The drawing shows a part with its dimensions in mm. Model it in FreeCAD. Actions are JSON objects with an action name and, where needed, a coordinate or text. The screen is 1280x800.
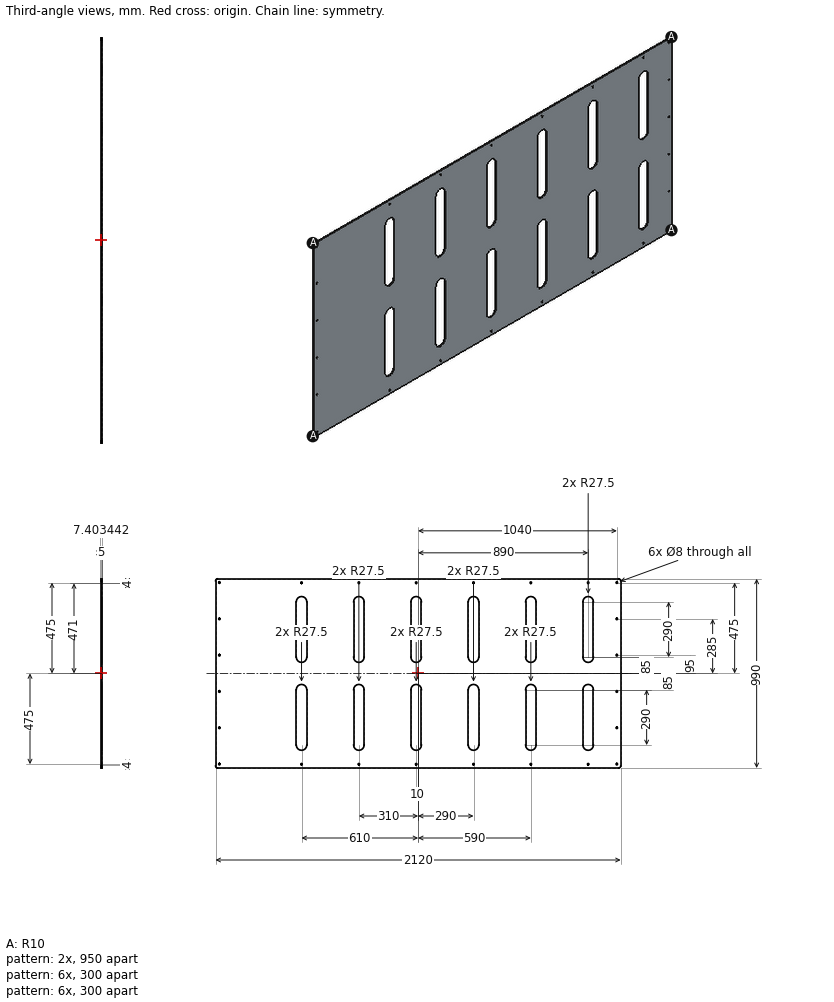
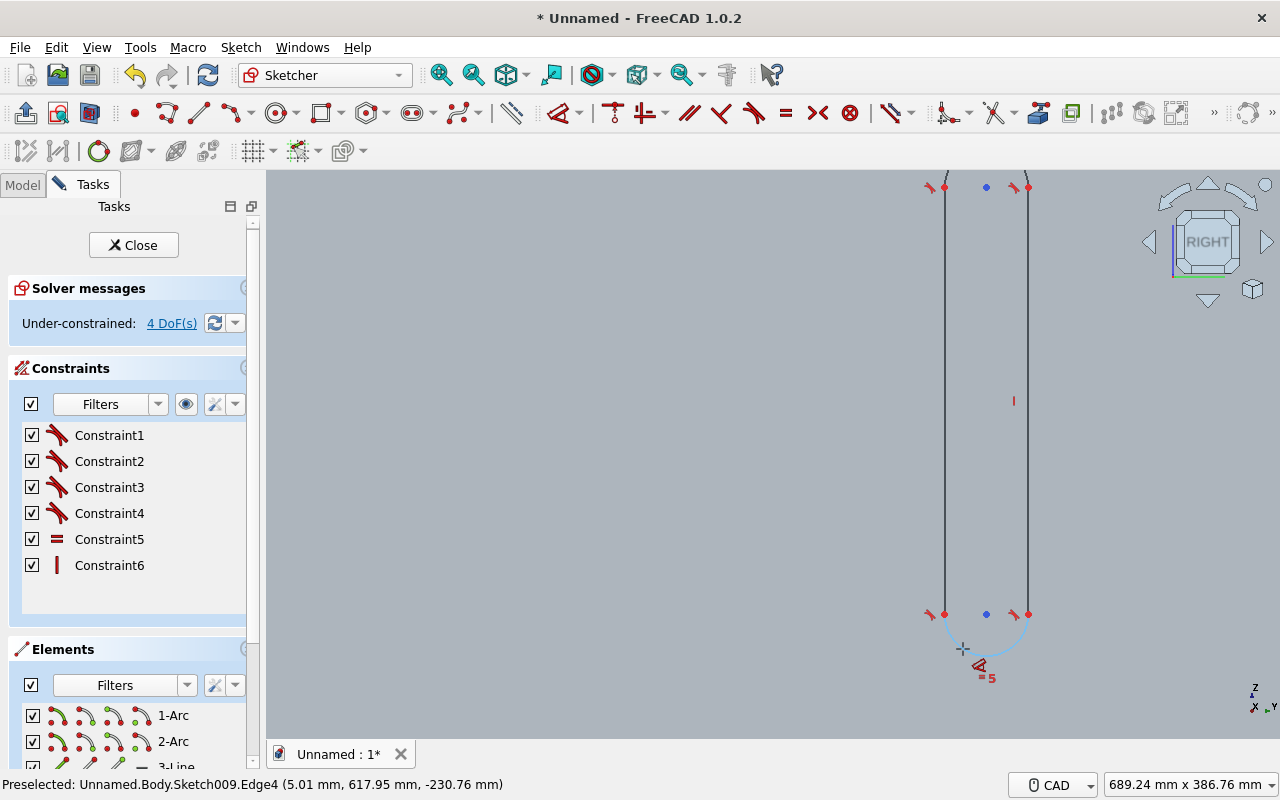
{"action": "left_click", "coordinate": [962, 648]}
{"action": "left_click", "coordinate": [943, 674]}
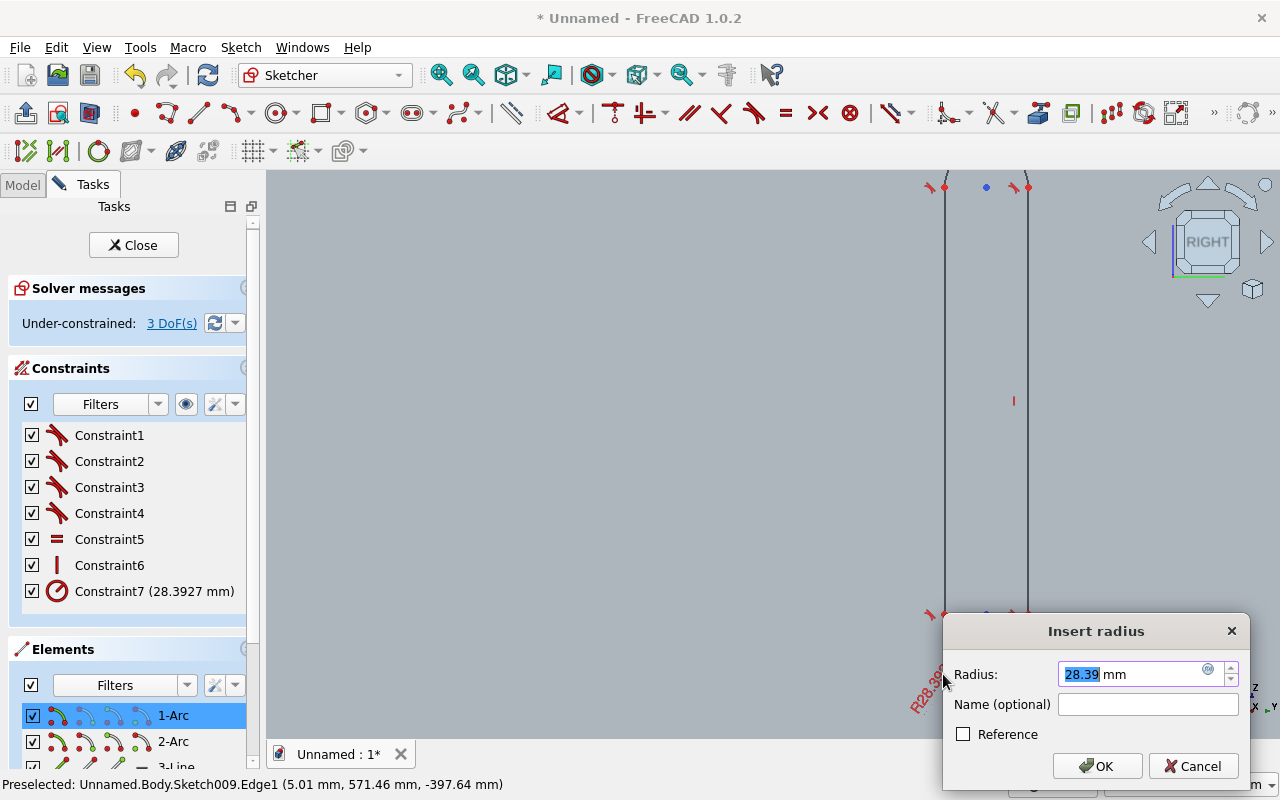
{"action": "type", "text": "27.5"}
{"action": "key", "text": "Return"}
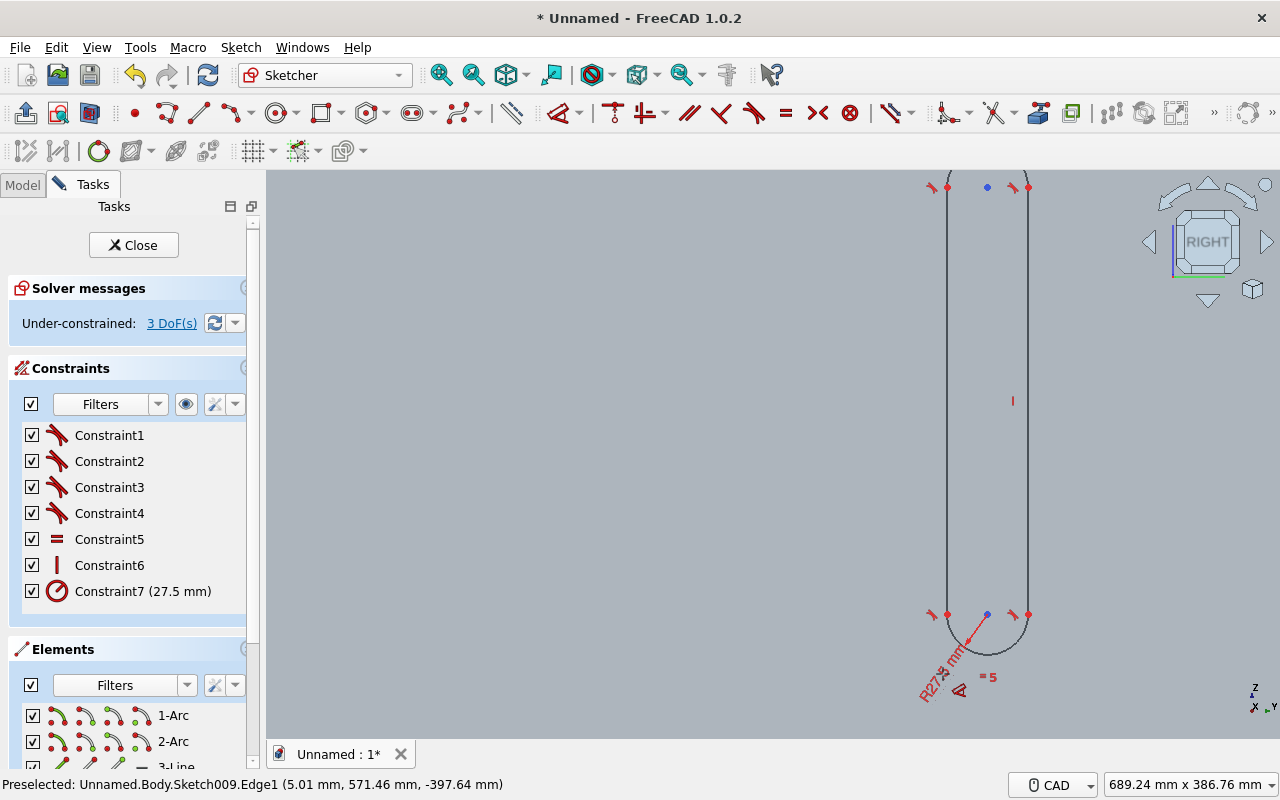
{"action": "left_click", "coordinate": [947, 486]}
{"action": "left_click", "coordinate": [981, 406]}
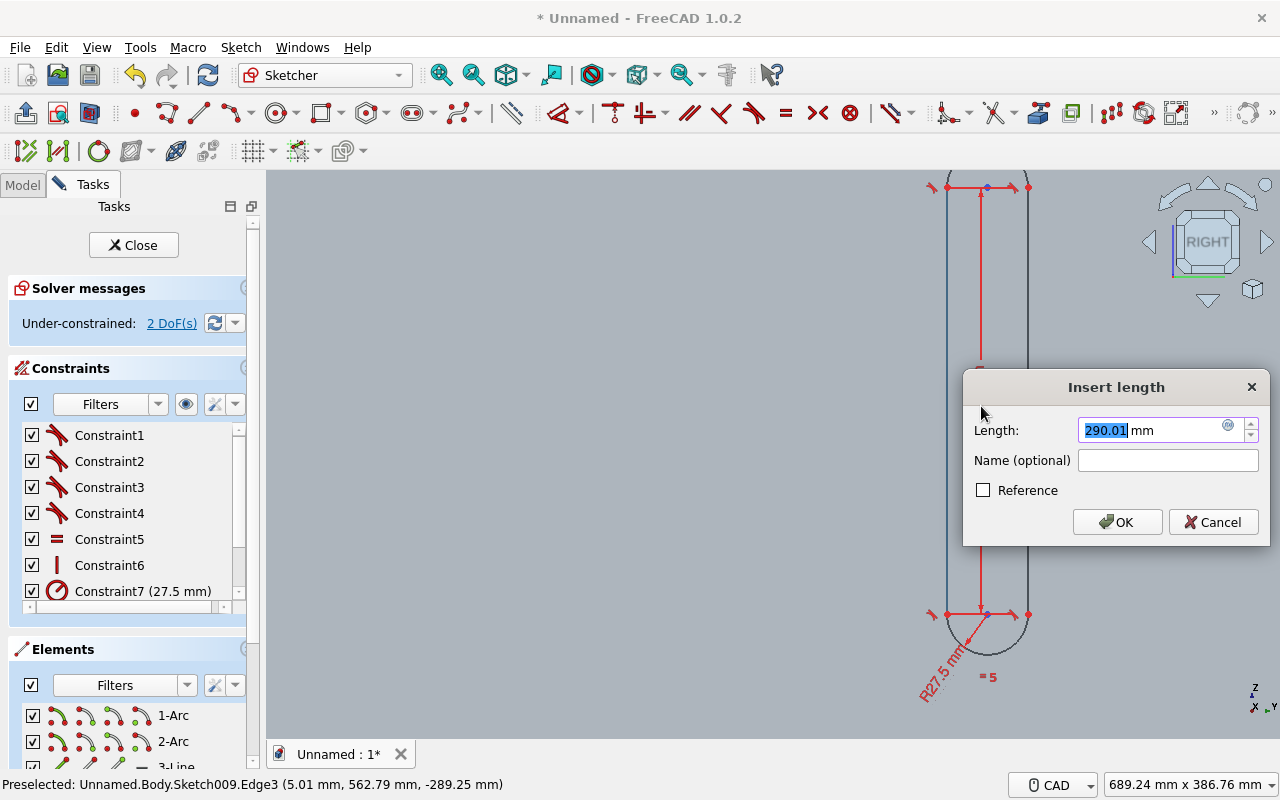
{"action": "type", "text": "290"}
{"action": "key", "text": "Return"}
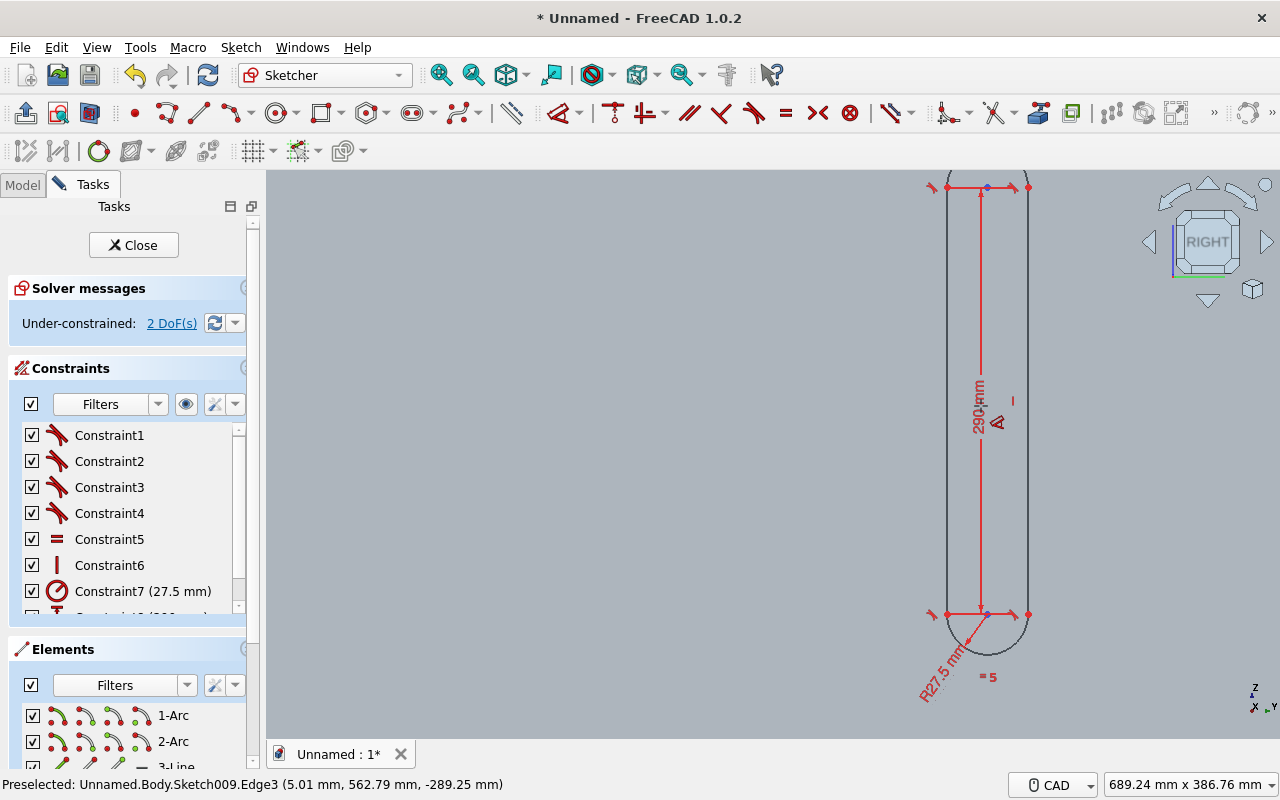
{"action": "scroll", "coordinate": [971, 652], "scroll_direction": "down", "scroll_amount": 2}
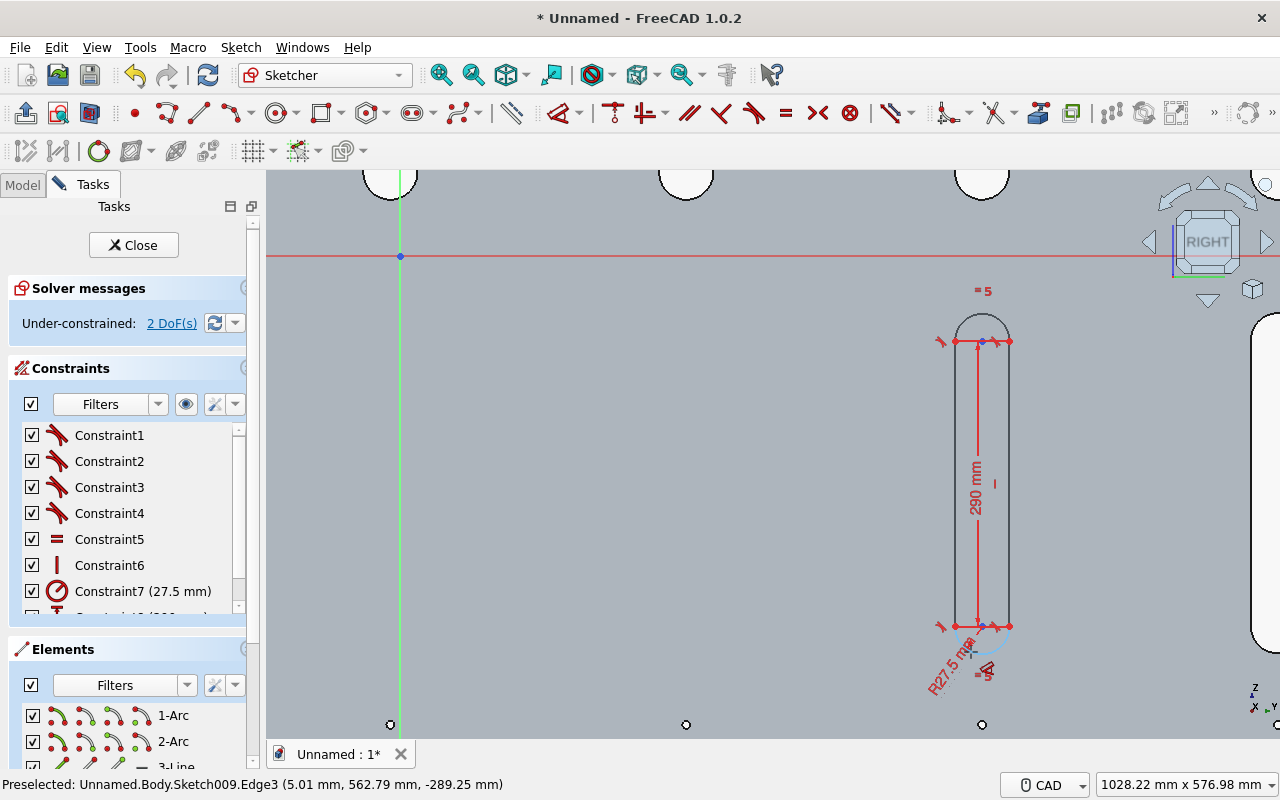
{"action": "left_click", "coordinate": [1009, 341]}
{"action": "left_click", "coordinate": [1043, 299]}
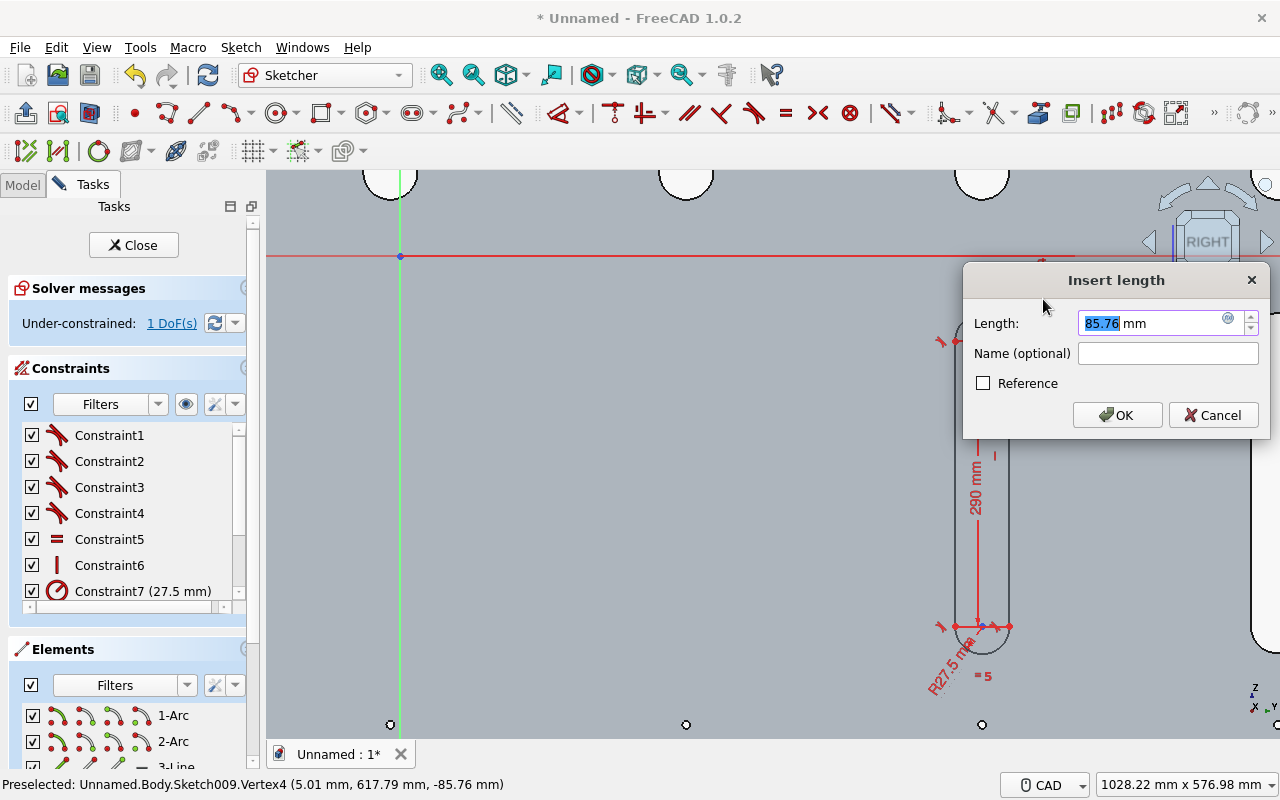
{"action": "type", "text": "85"}
{"action": "key", "text": "Return"}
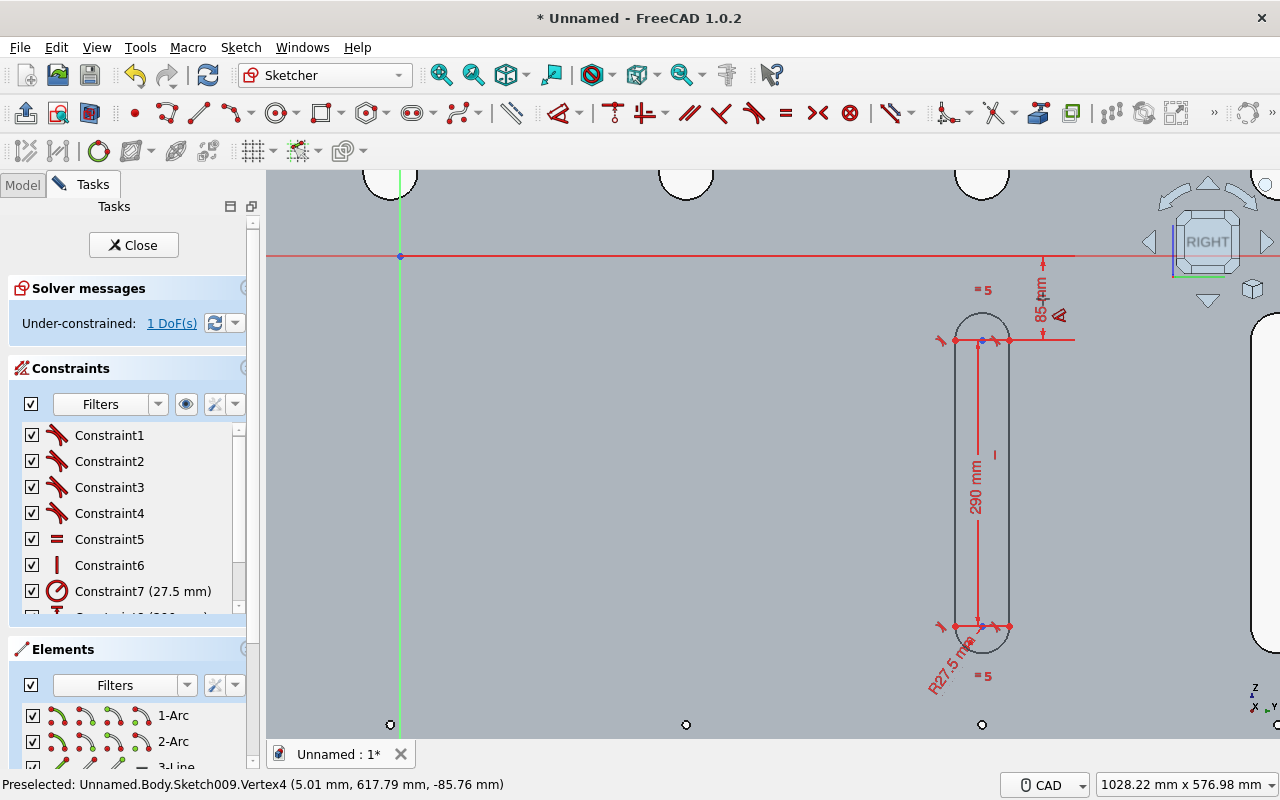
{"action": "left_click", "coordinate": [982, 626]}
{"action": "left_click", "coordinate": [691, 222]}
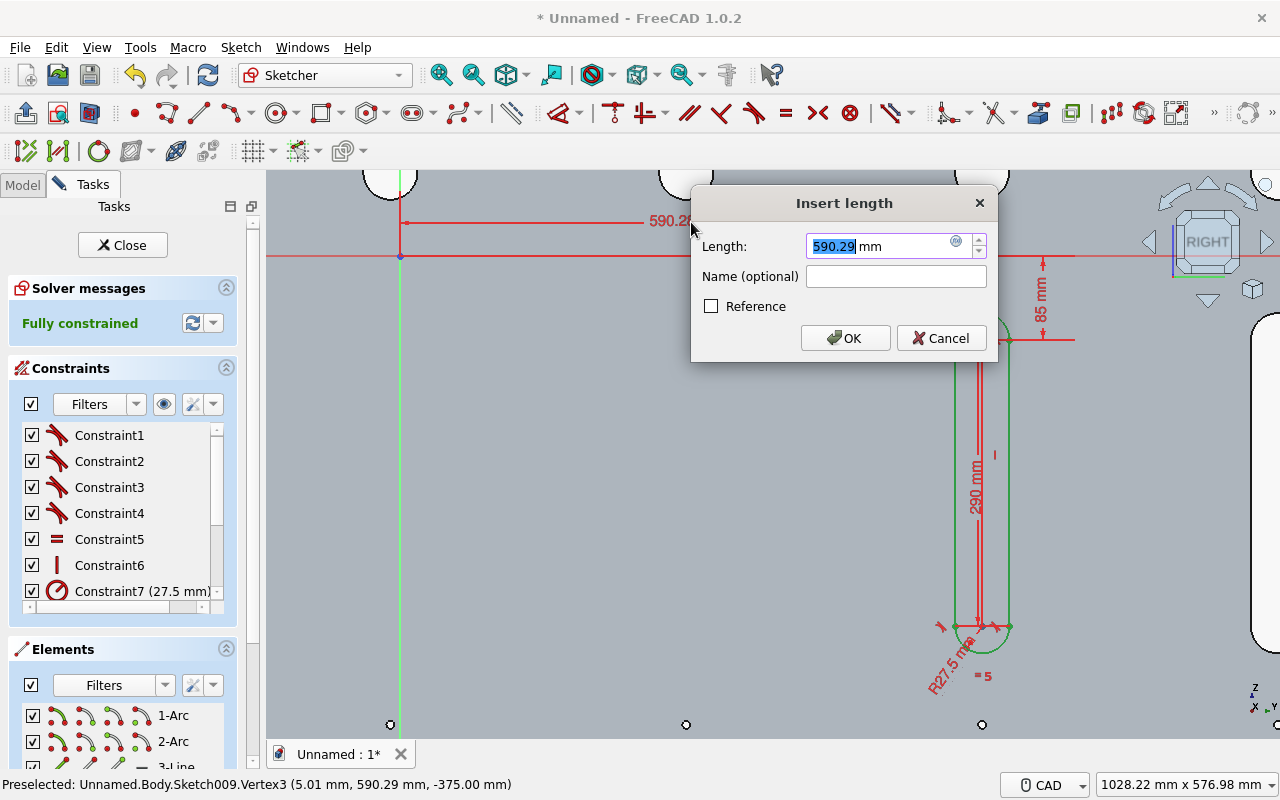
{"action": "type", "text": "590"}
{"action": "key", "text": "Return"}
{"action": "key", "text": "Escape"}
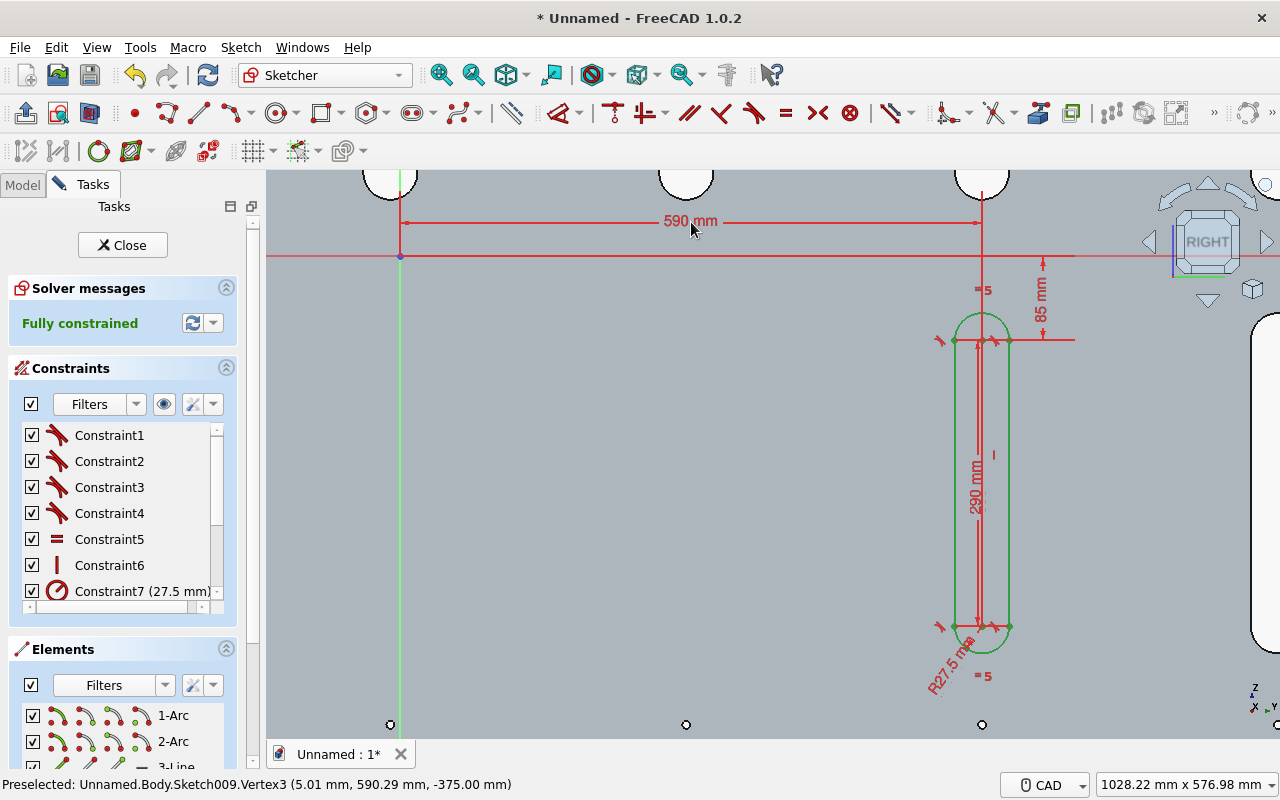
{"action": "left_click", "coordinate": [123, 245]}